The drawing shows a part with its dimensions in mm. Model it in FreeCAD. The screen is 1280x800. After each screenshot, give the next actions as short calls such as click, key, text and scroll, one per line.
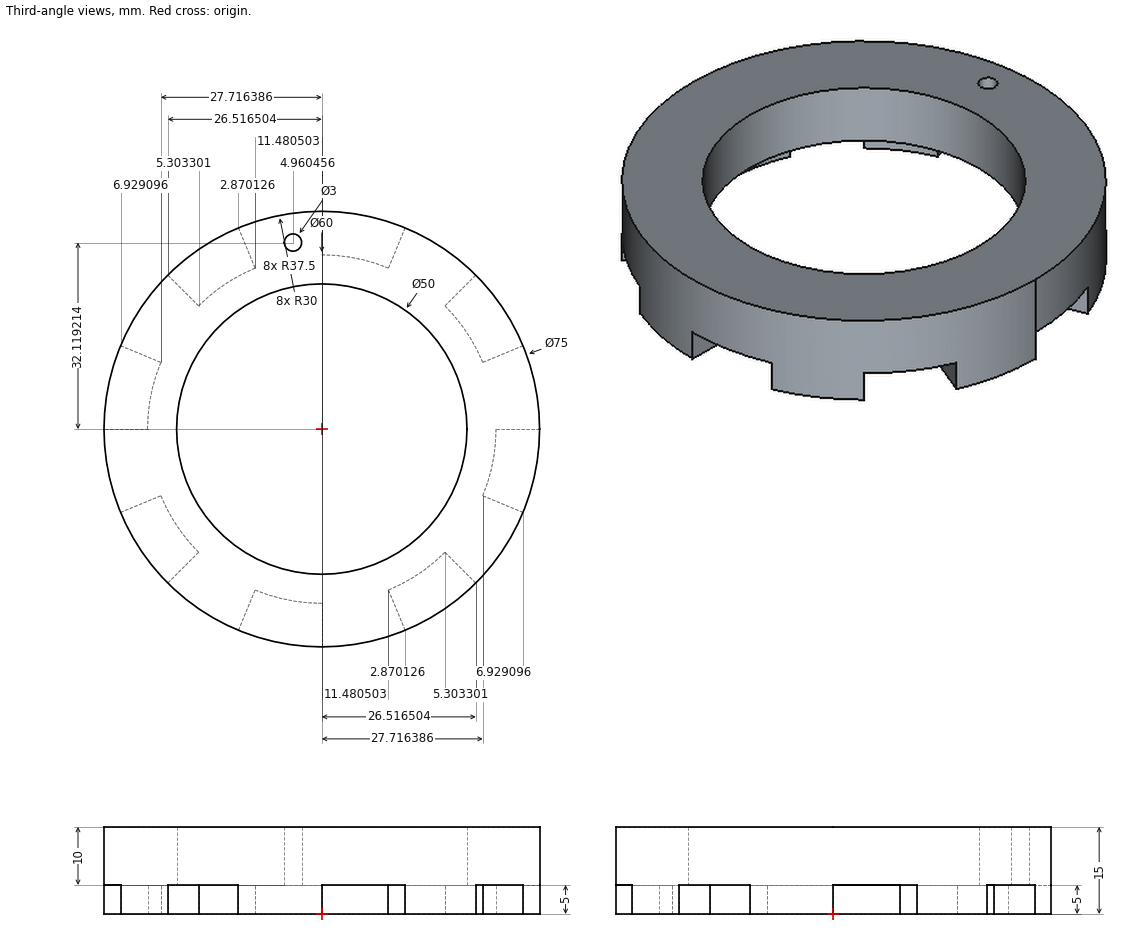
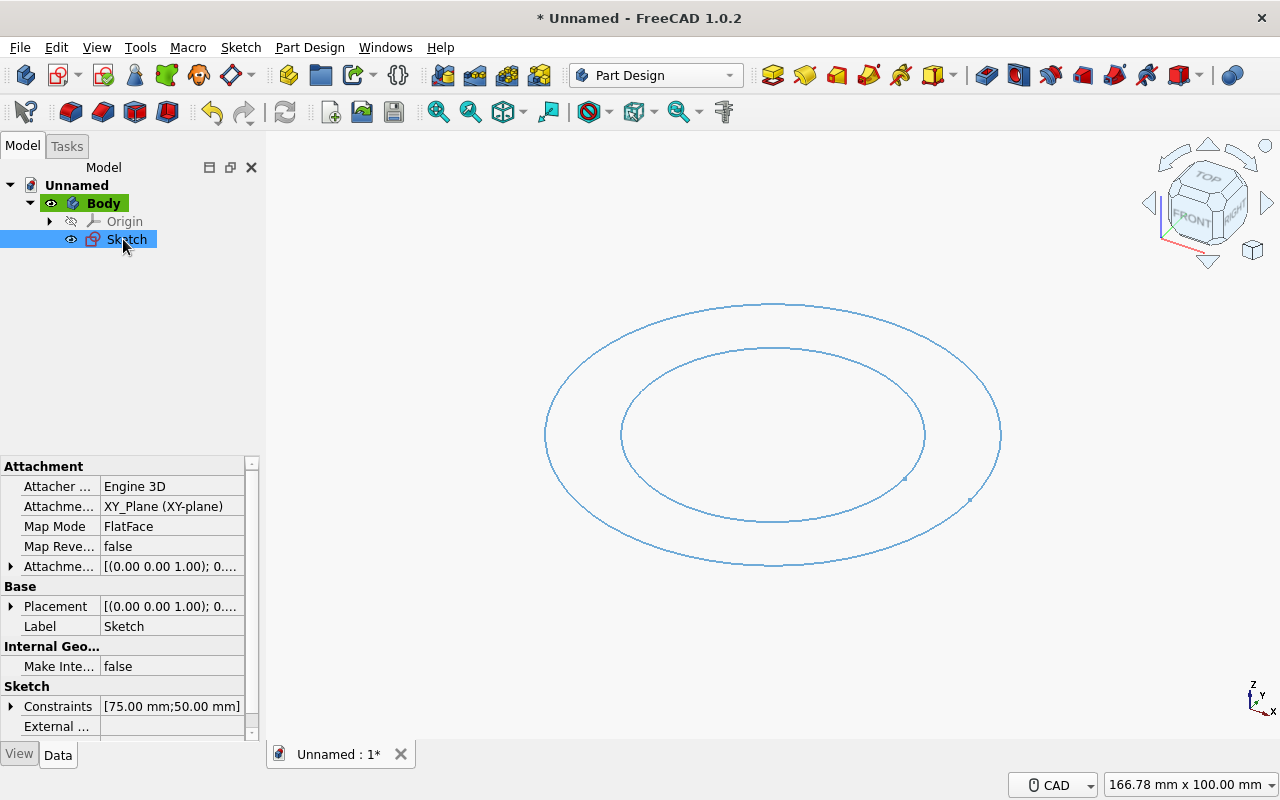
click(774, 76)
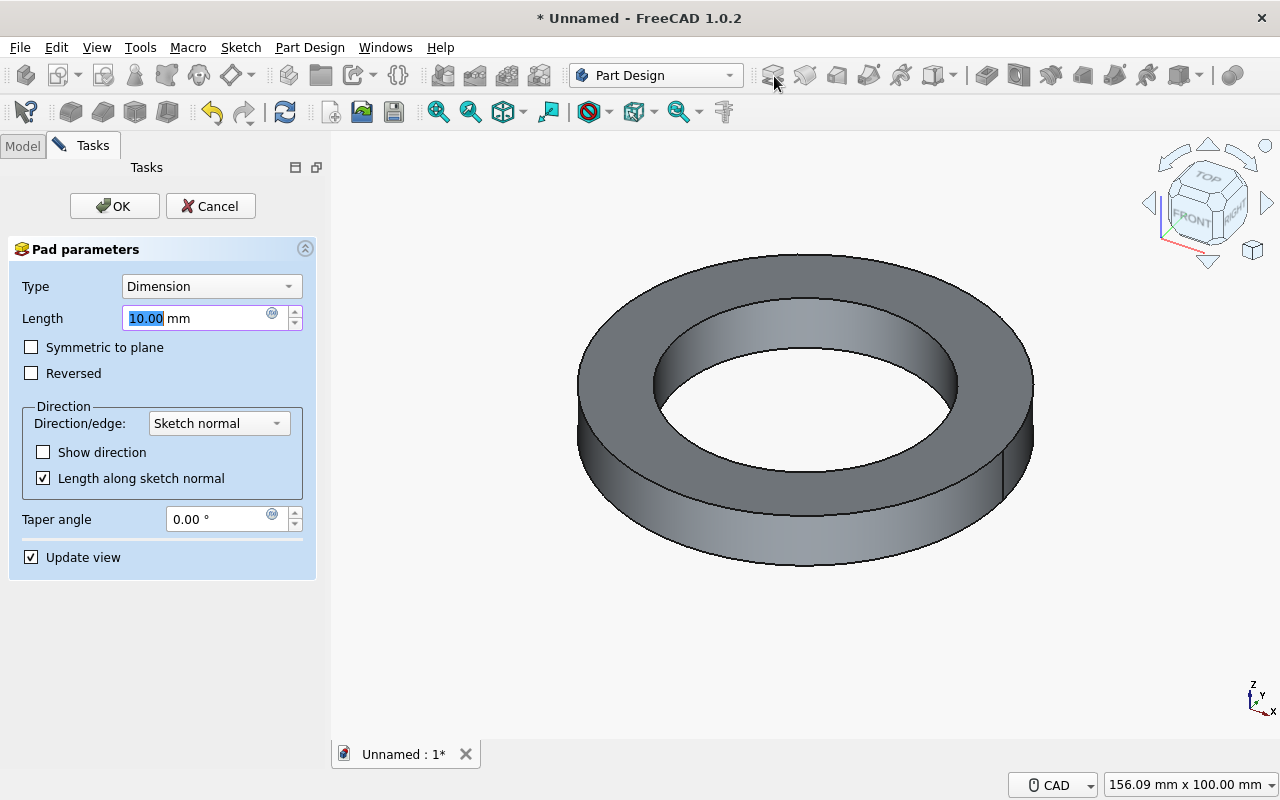
text(15)
key(Tab)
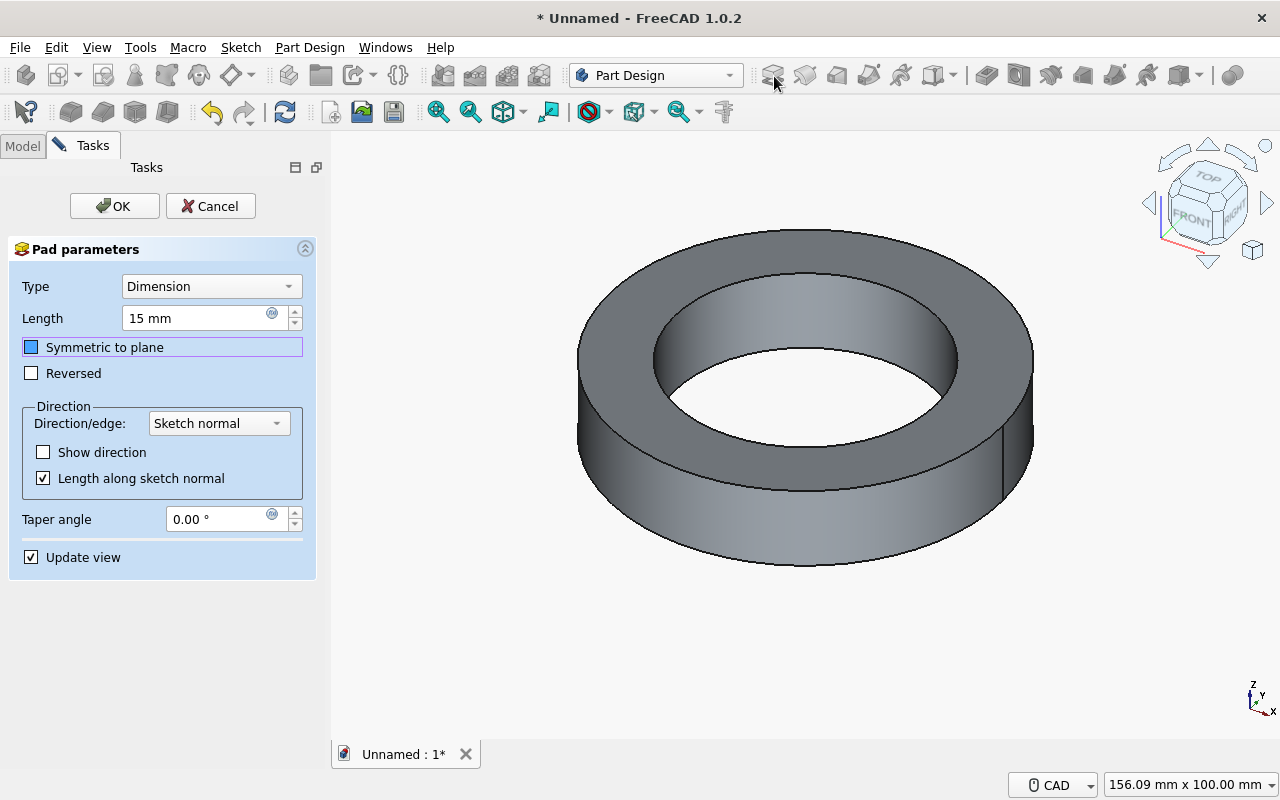
click(115, 206)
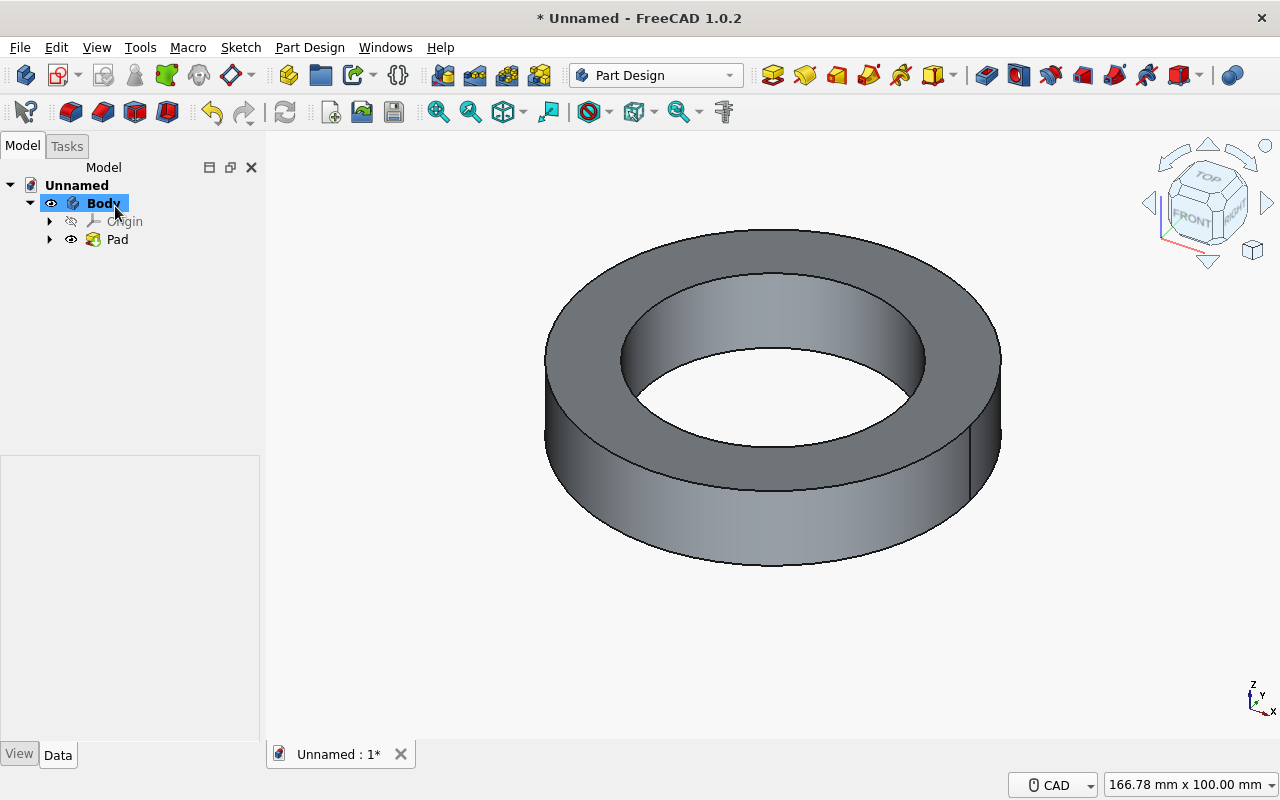
click(58, 76)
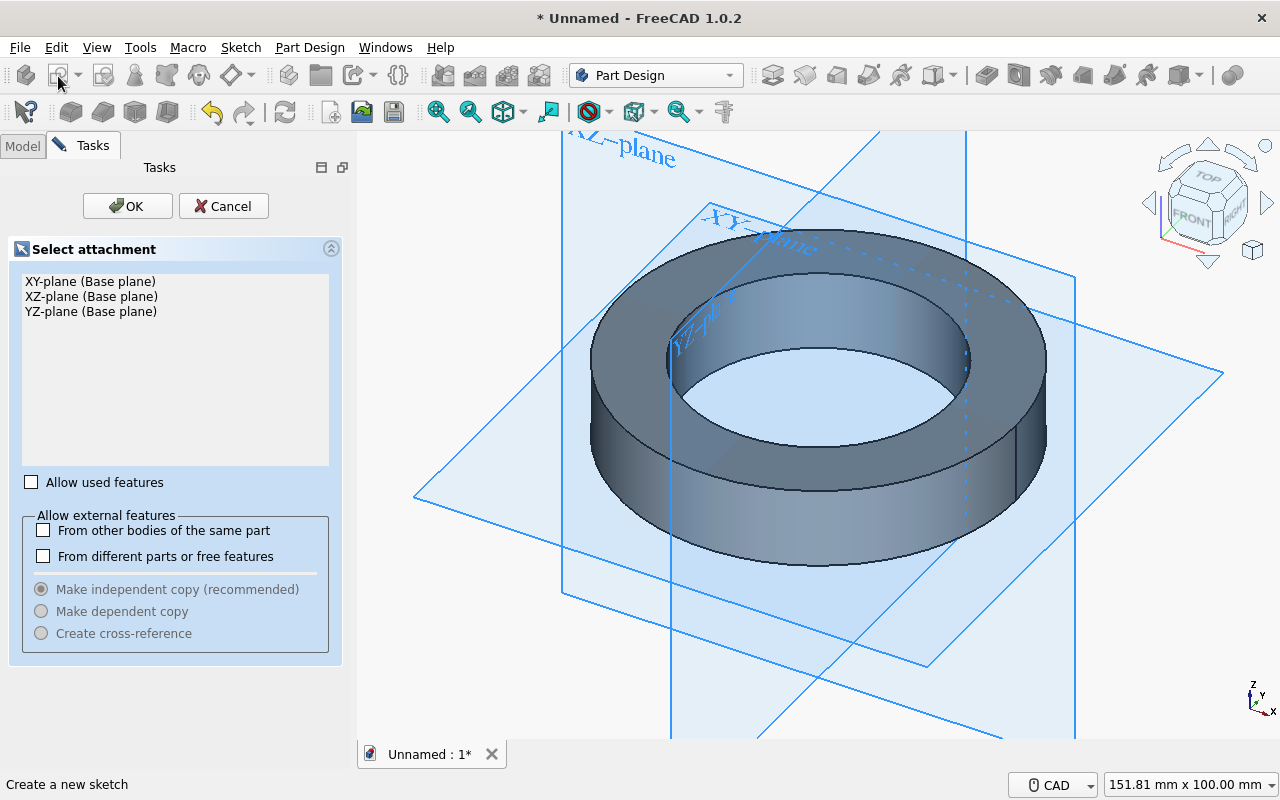
click(82, 282)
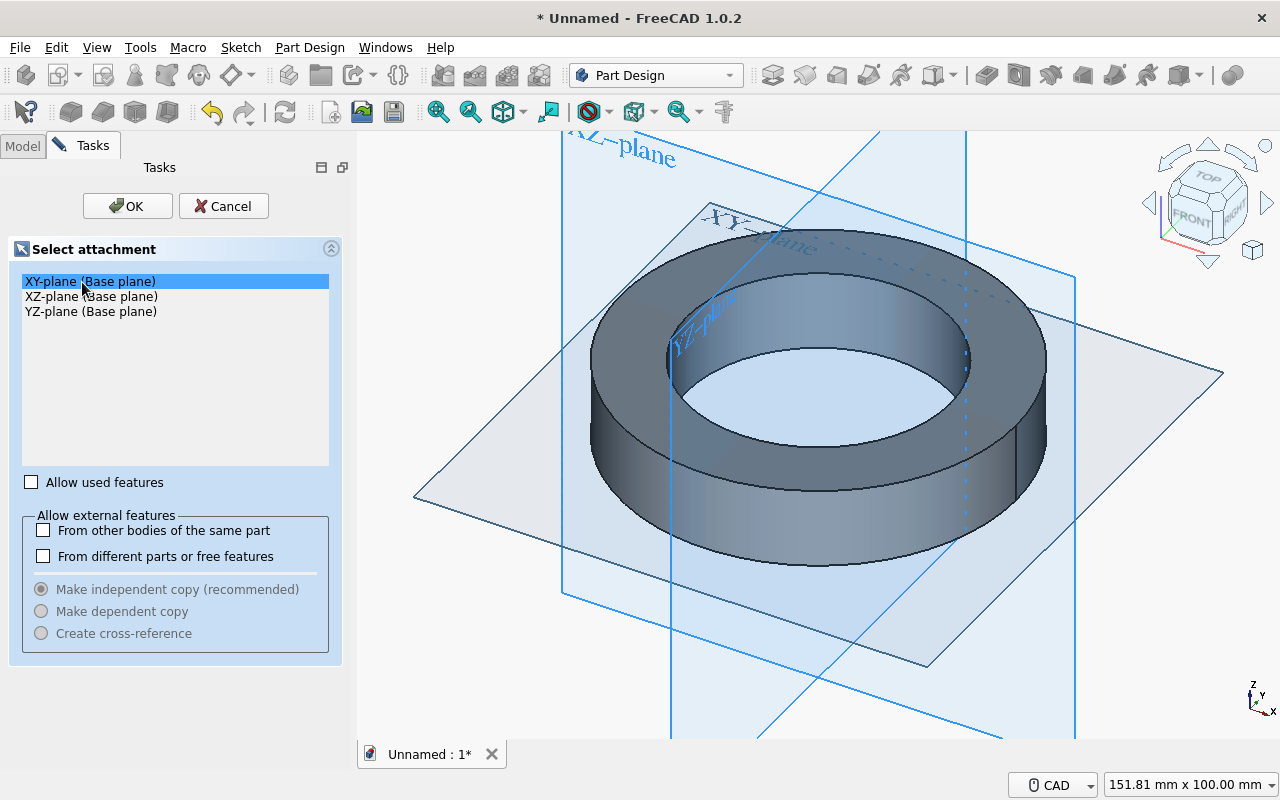
click(128, 206)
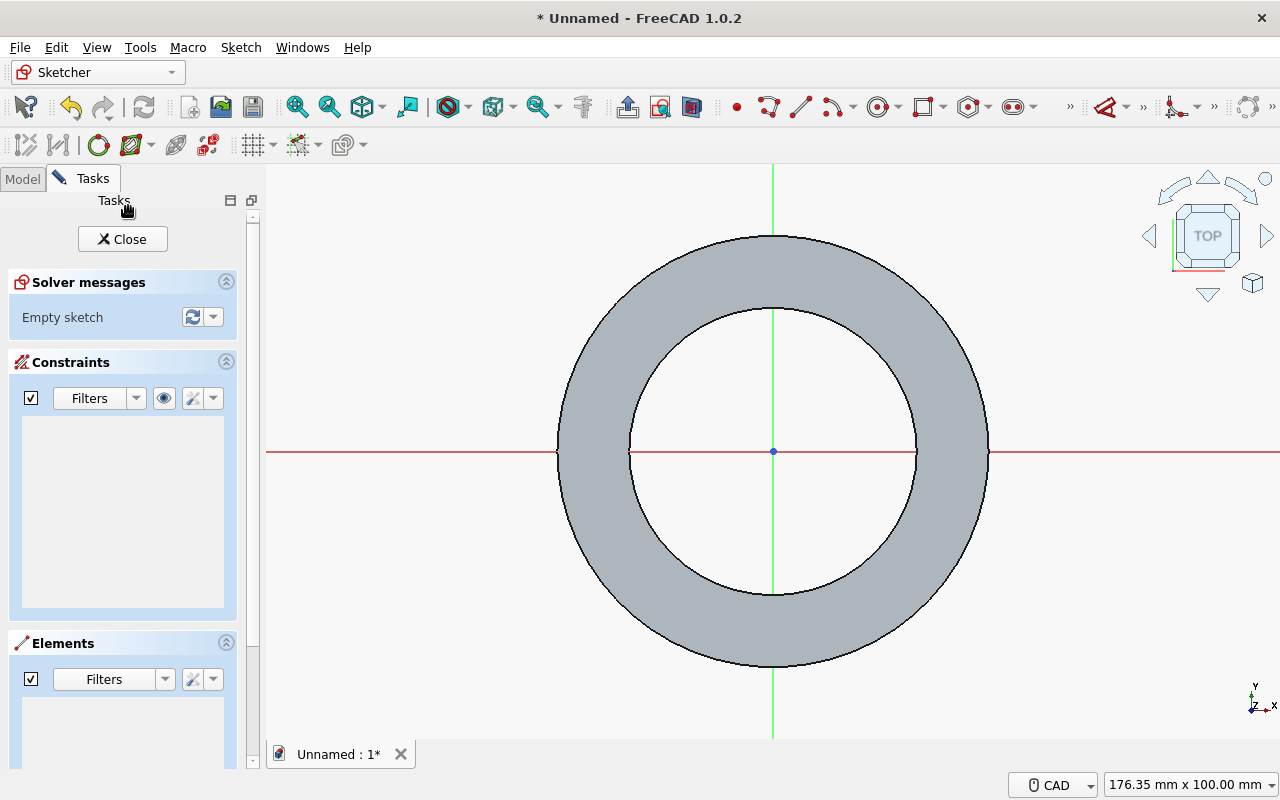
key(q)
key(s)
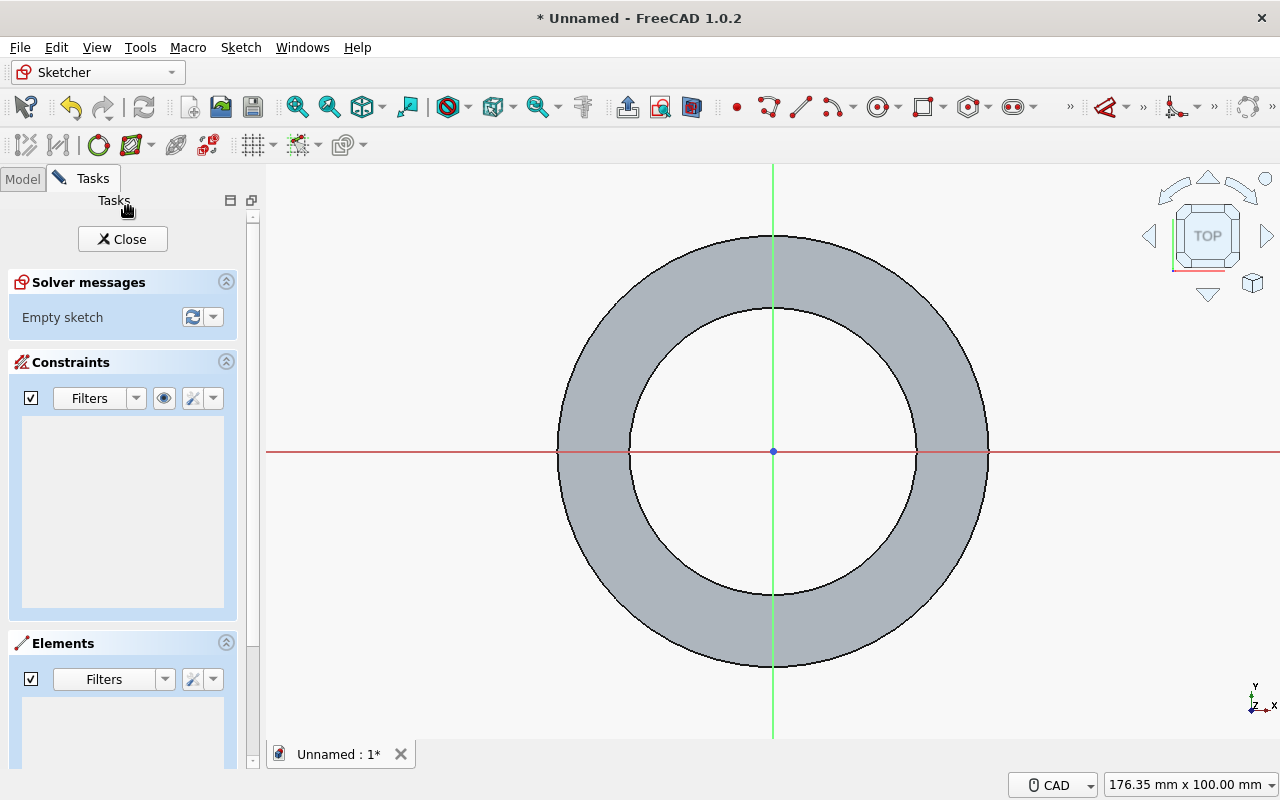
key(g)
key(c)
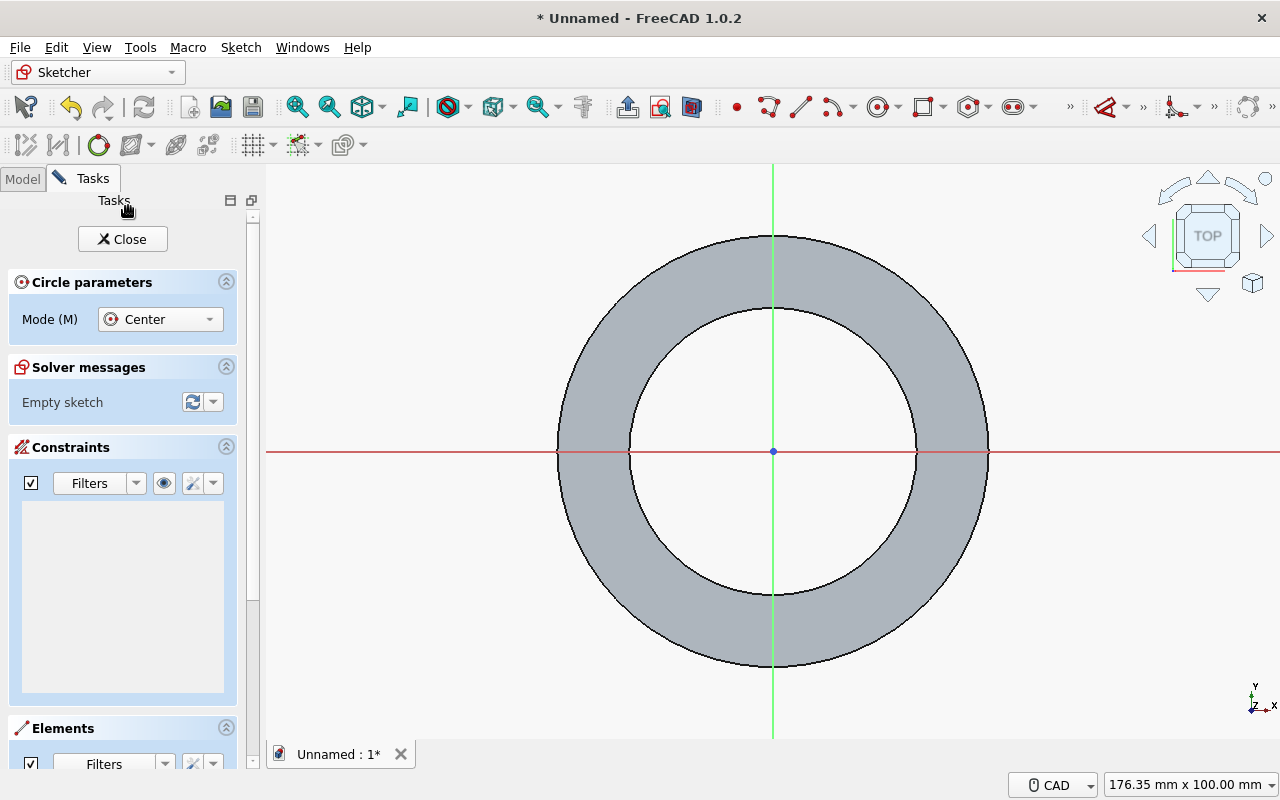
click(773, 452)
move(895, 330)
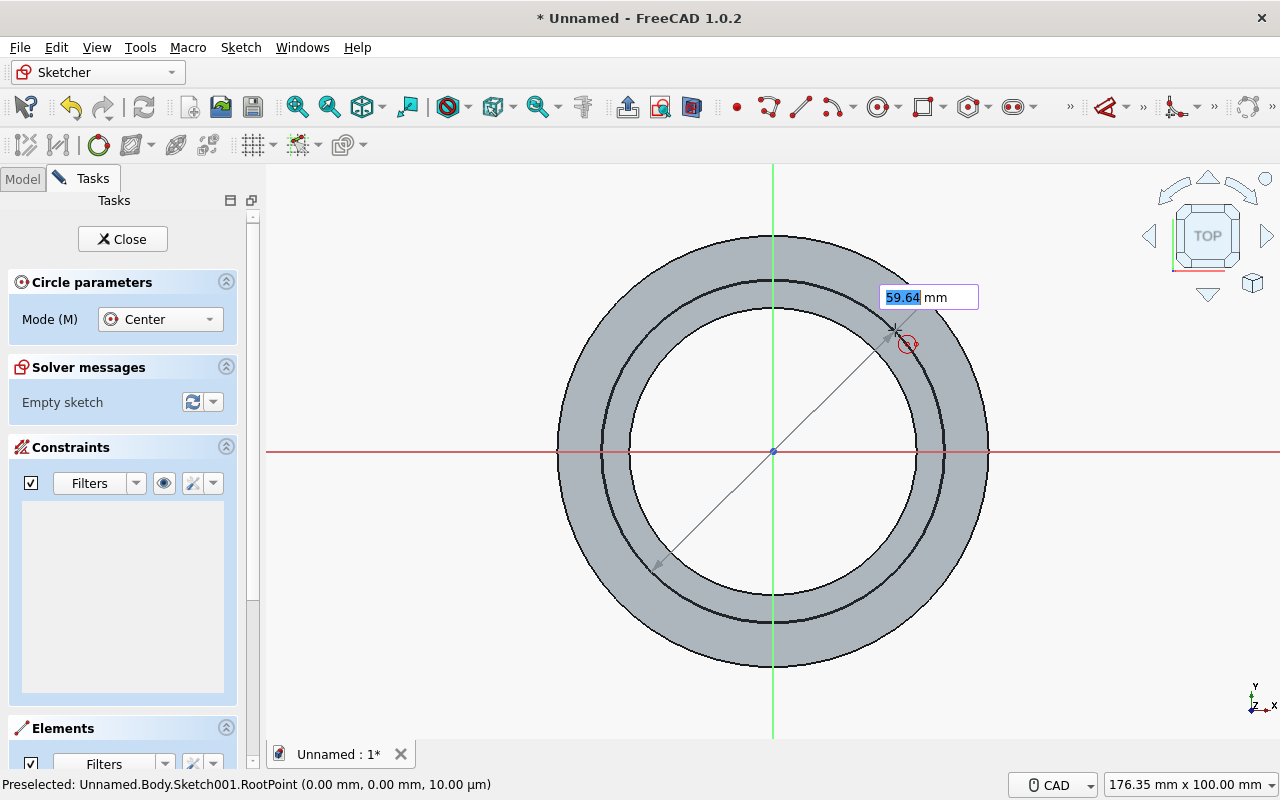
text(60)
key(Return)
key(Escape)